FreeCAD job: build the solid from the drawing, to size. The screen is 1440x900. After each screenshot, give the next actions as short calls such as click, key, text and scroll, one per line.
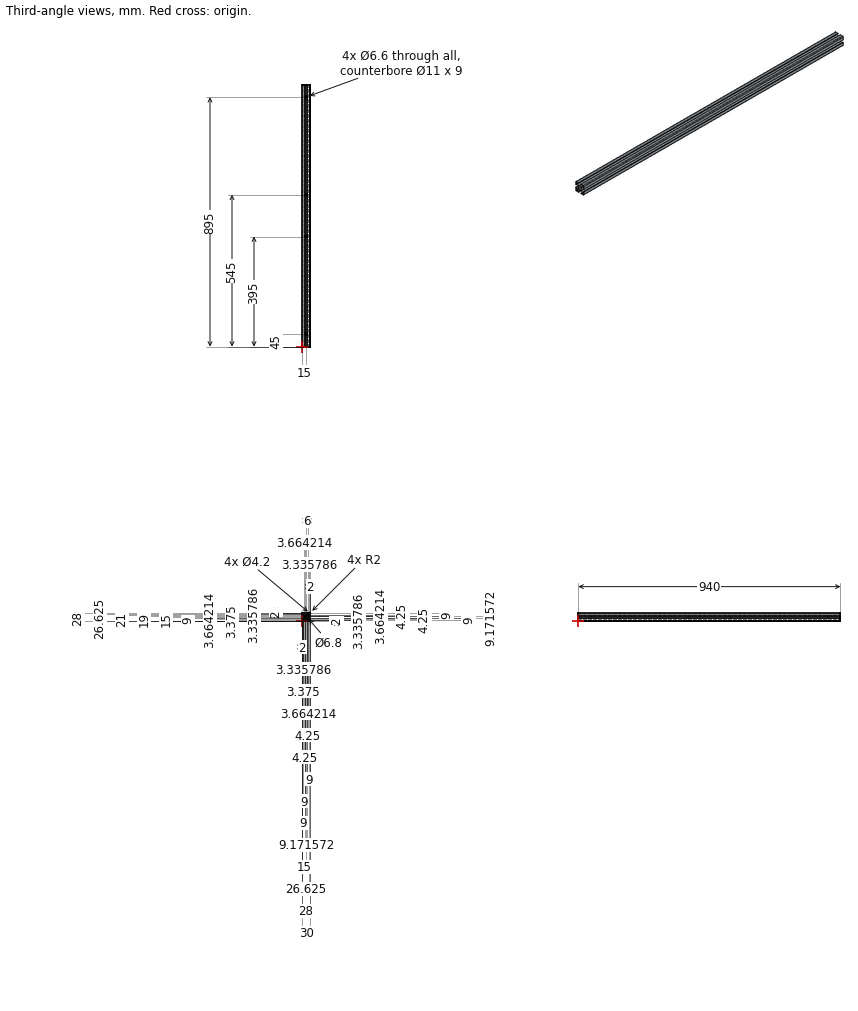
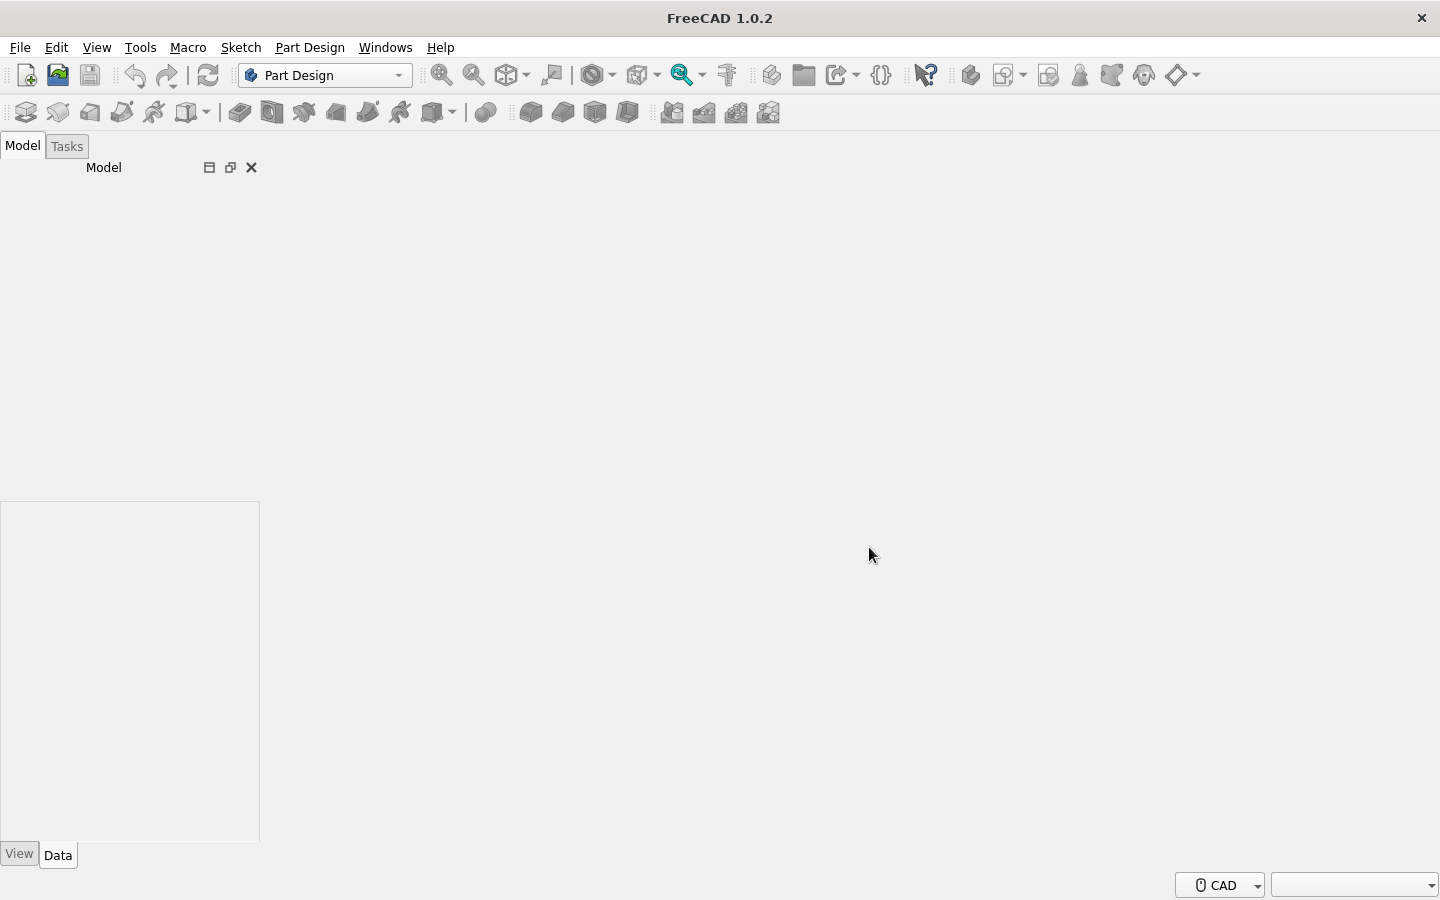
click(26, 76)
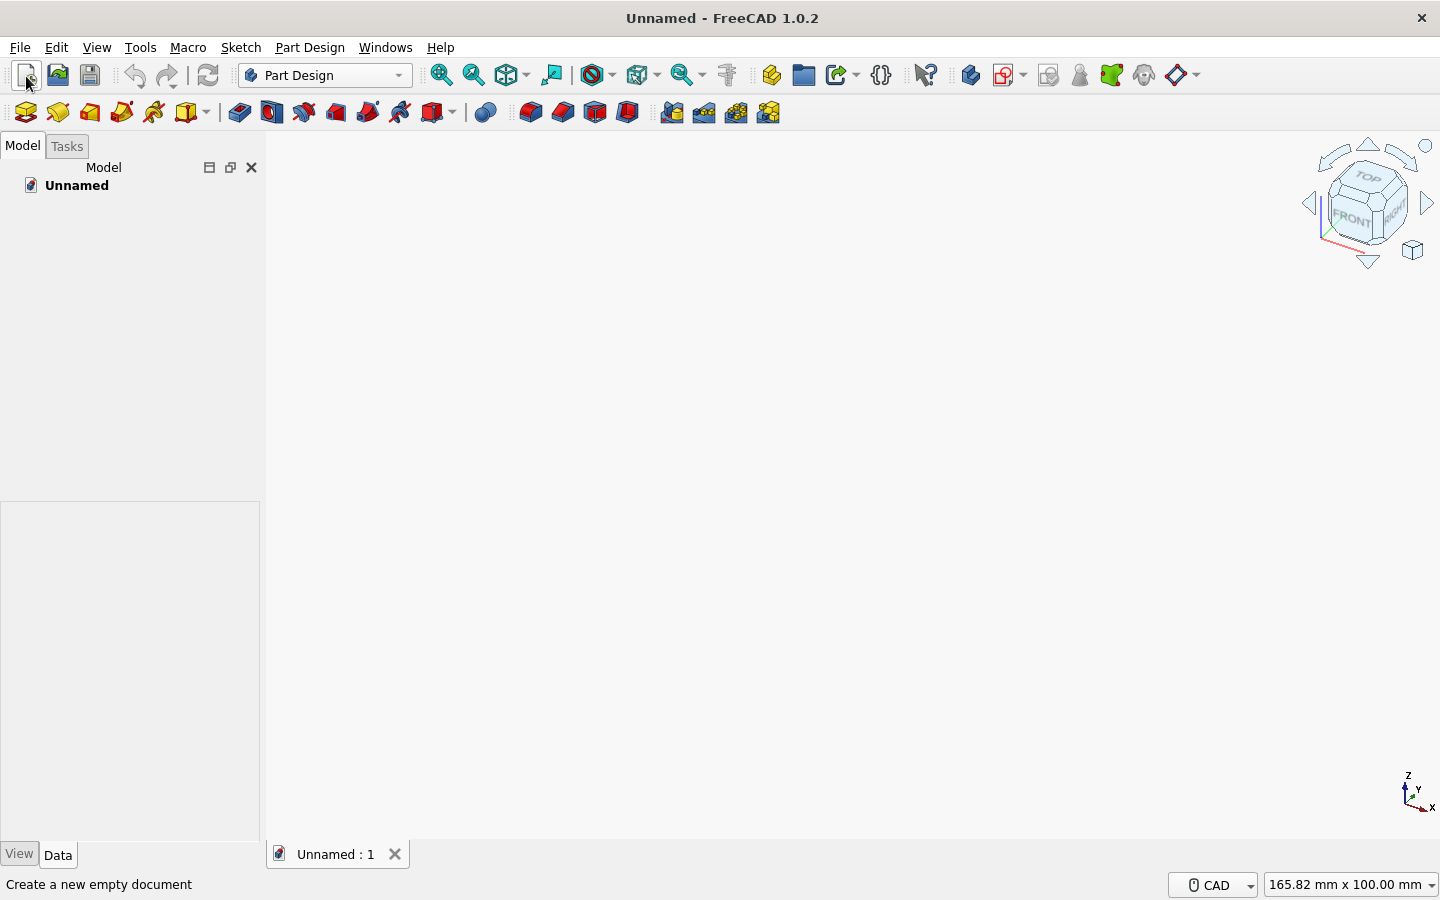
click(1004, 76)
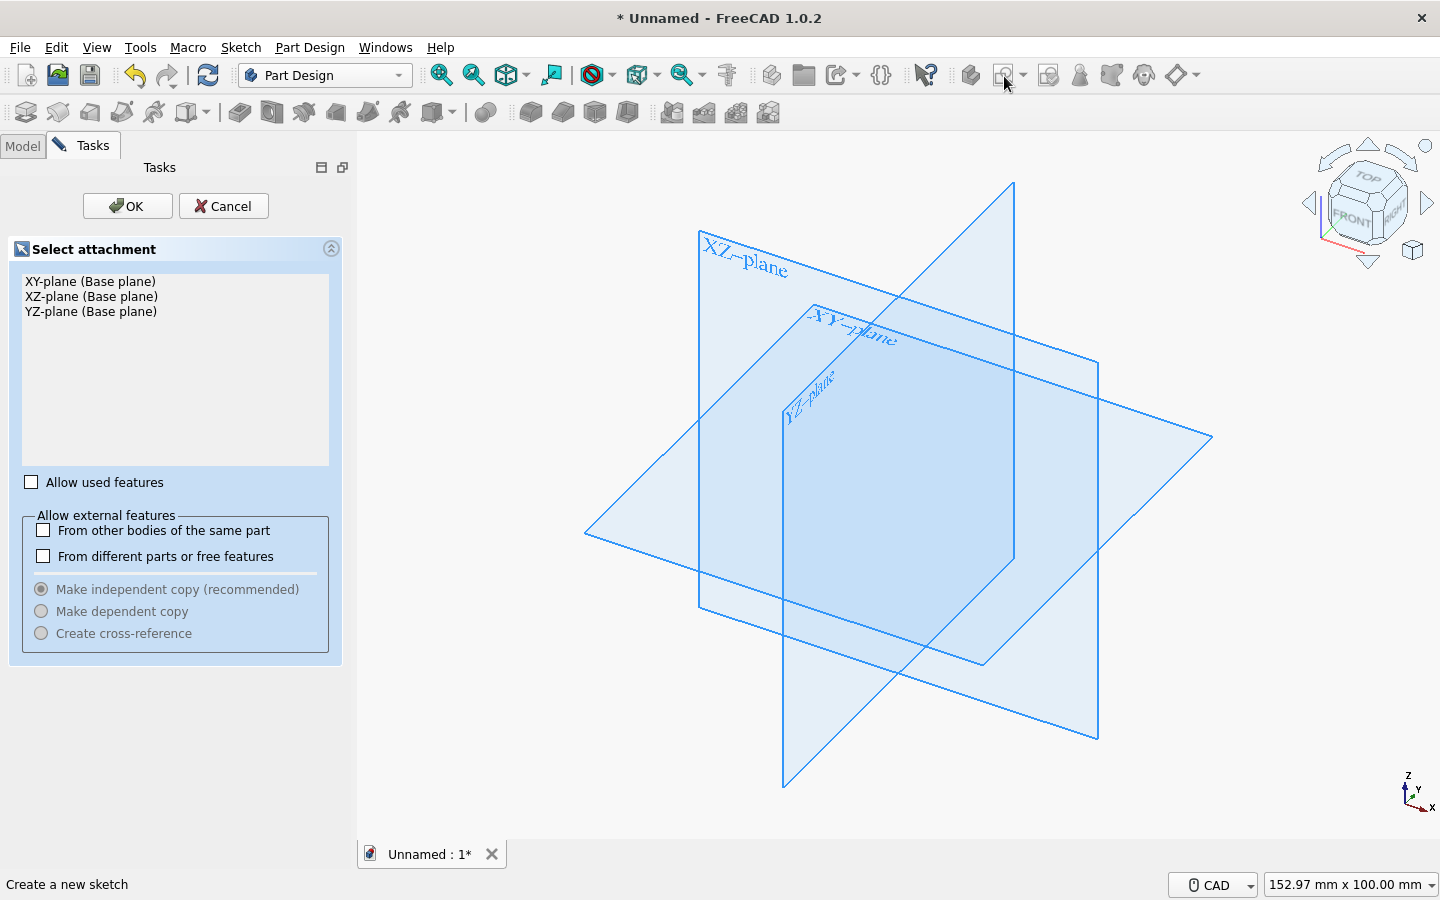
click(82, 296)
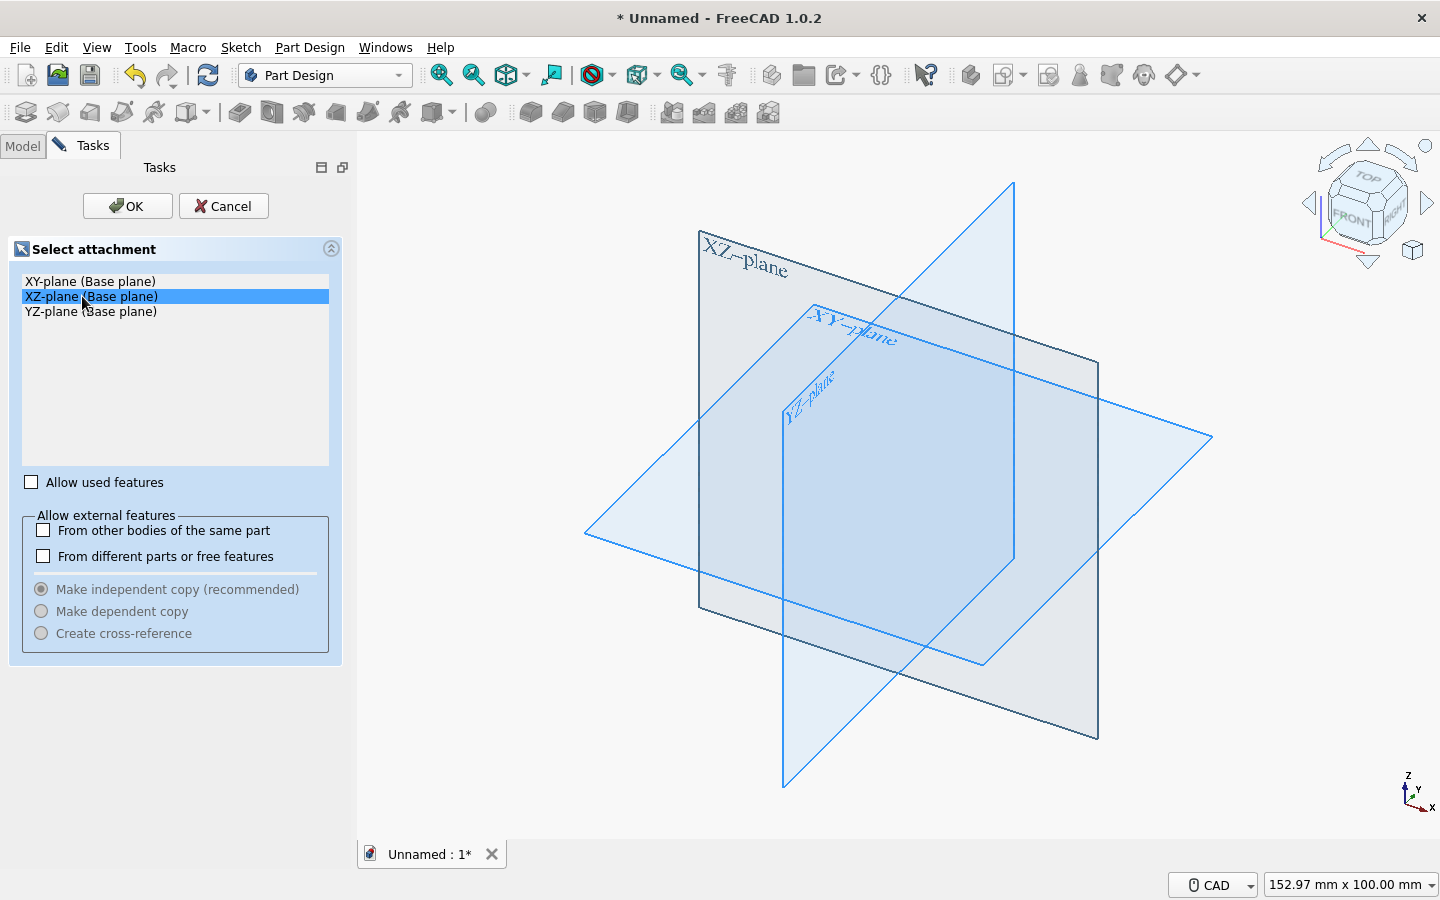
click(128, 206)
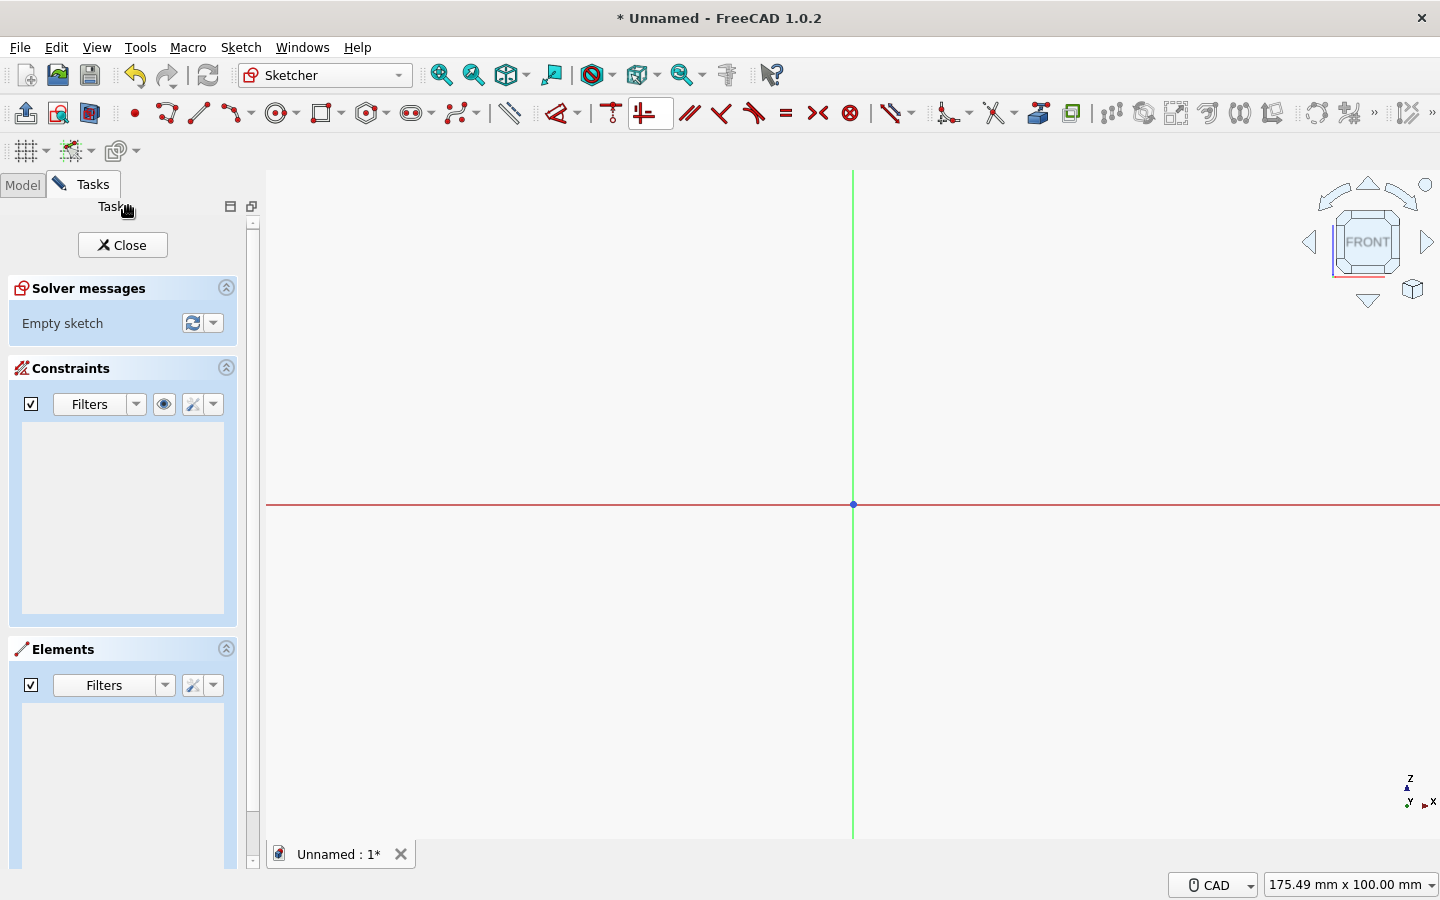
scroll(1091, 322, up, 4)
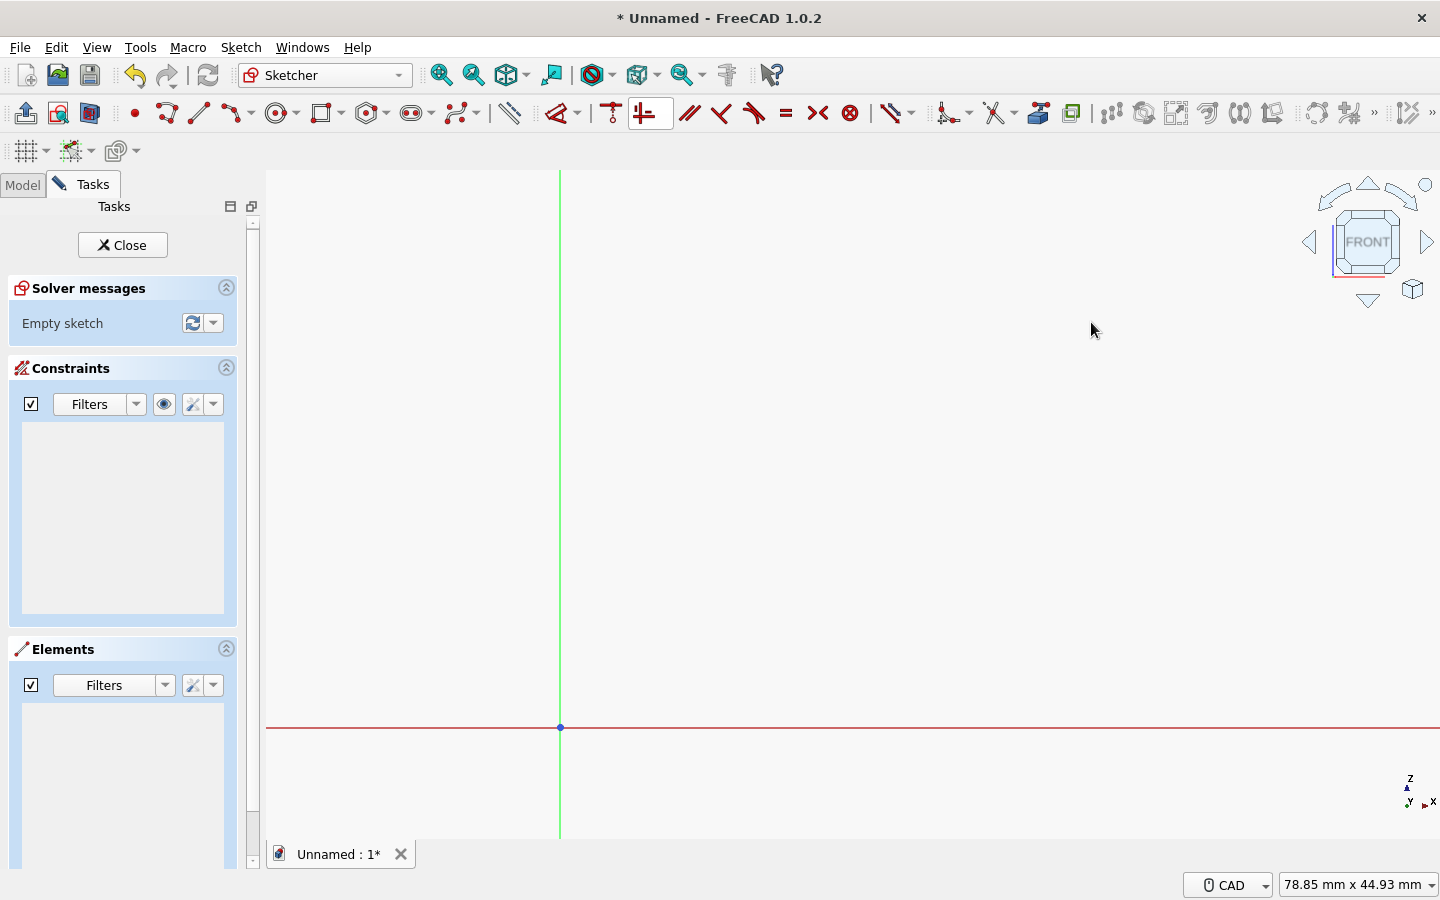
key(g)
key(m)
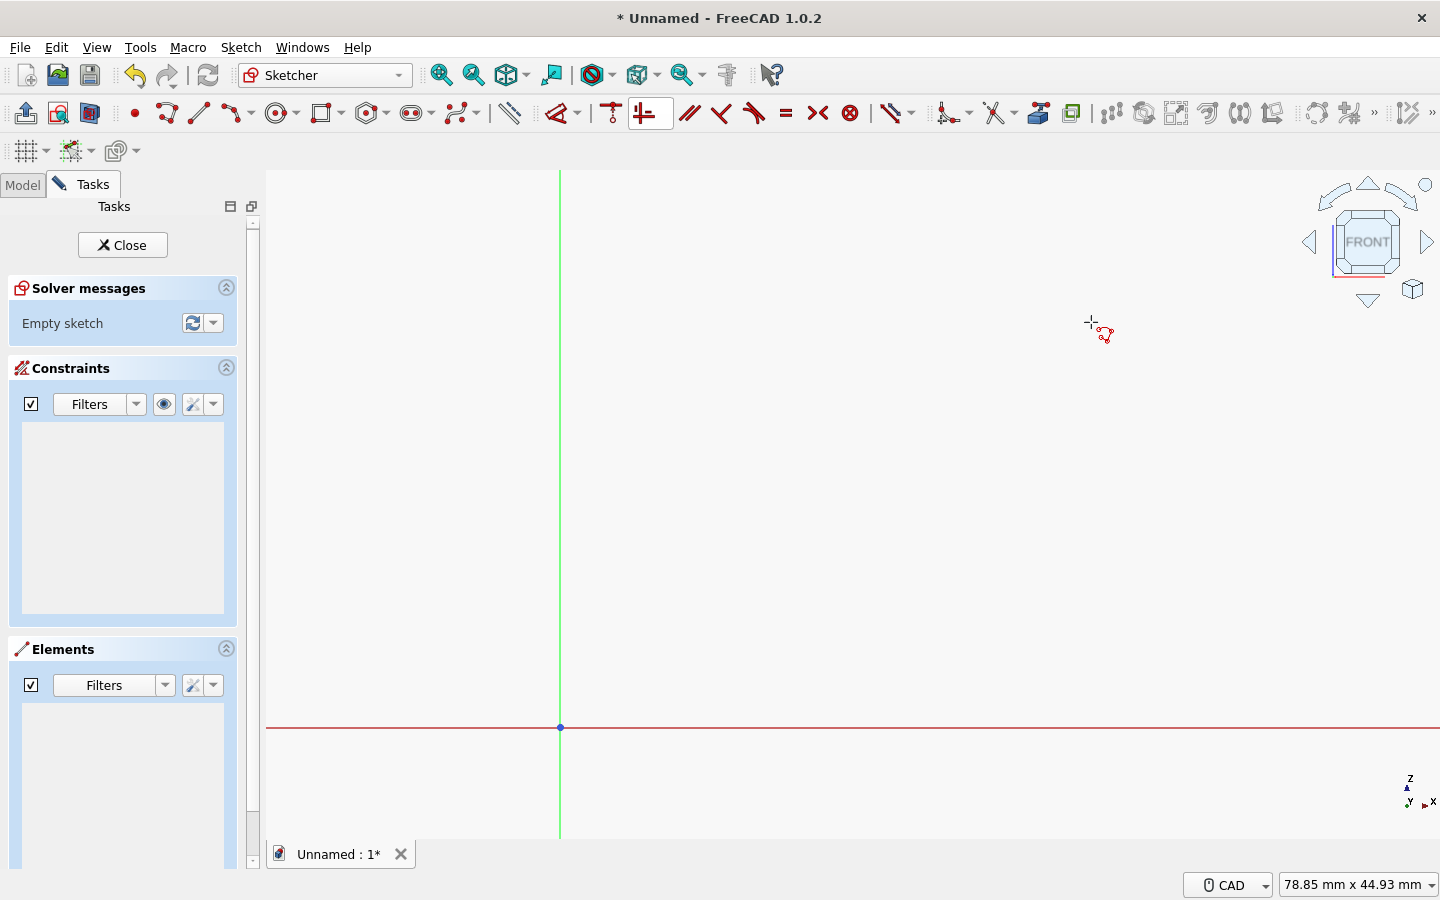
click(1007, 311)
click(1007, 445)
click(977, 445)
click(977, 382)
click(928, 382)
click(873, 436)
click(873, 573)
click(928, 627)
click(977, 627)
click(977, 564)
click(1007, 564)
click(1007, 698)
right_click(1007, 698)